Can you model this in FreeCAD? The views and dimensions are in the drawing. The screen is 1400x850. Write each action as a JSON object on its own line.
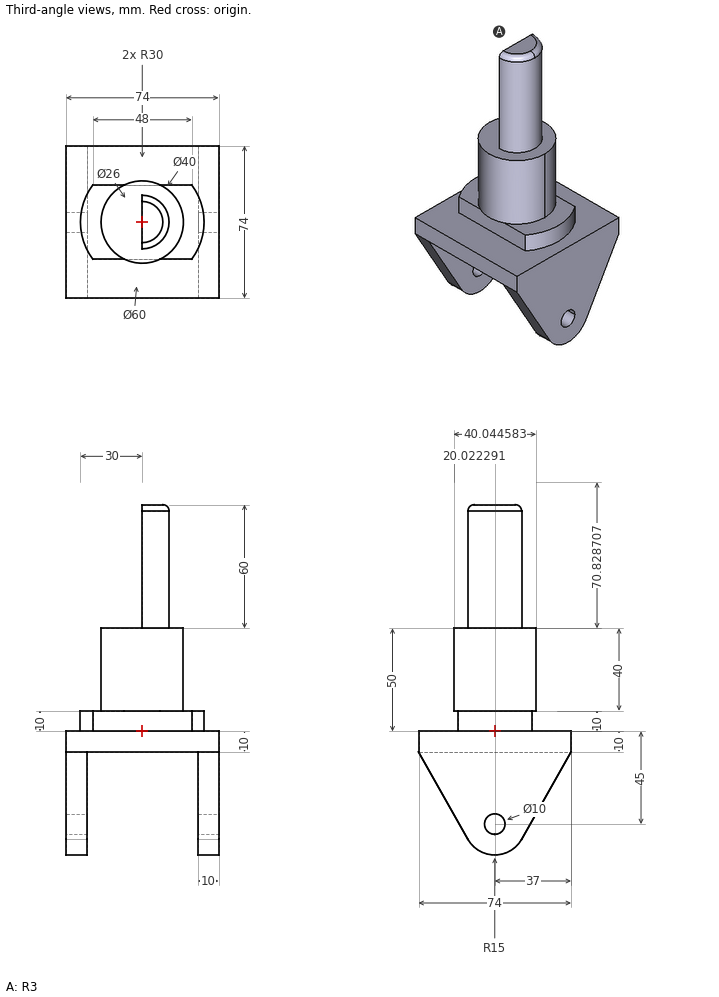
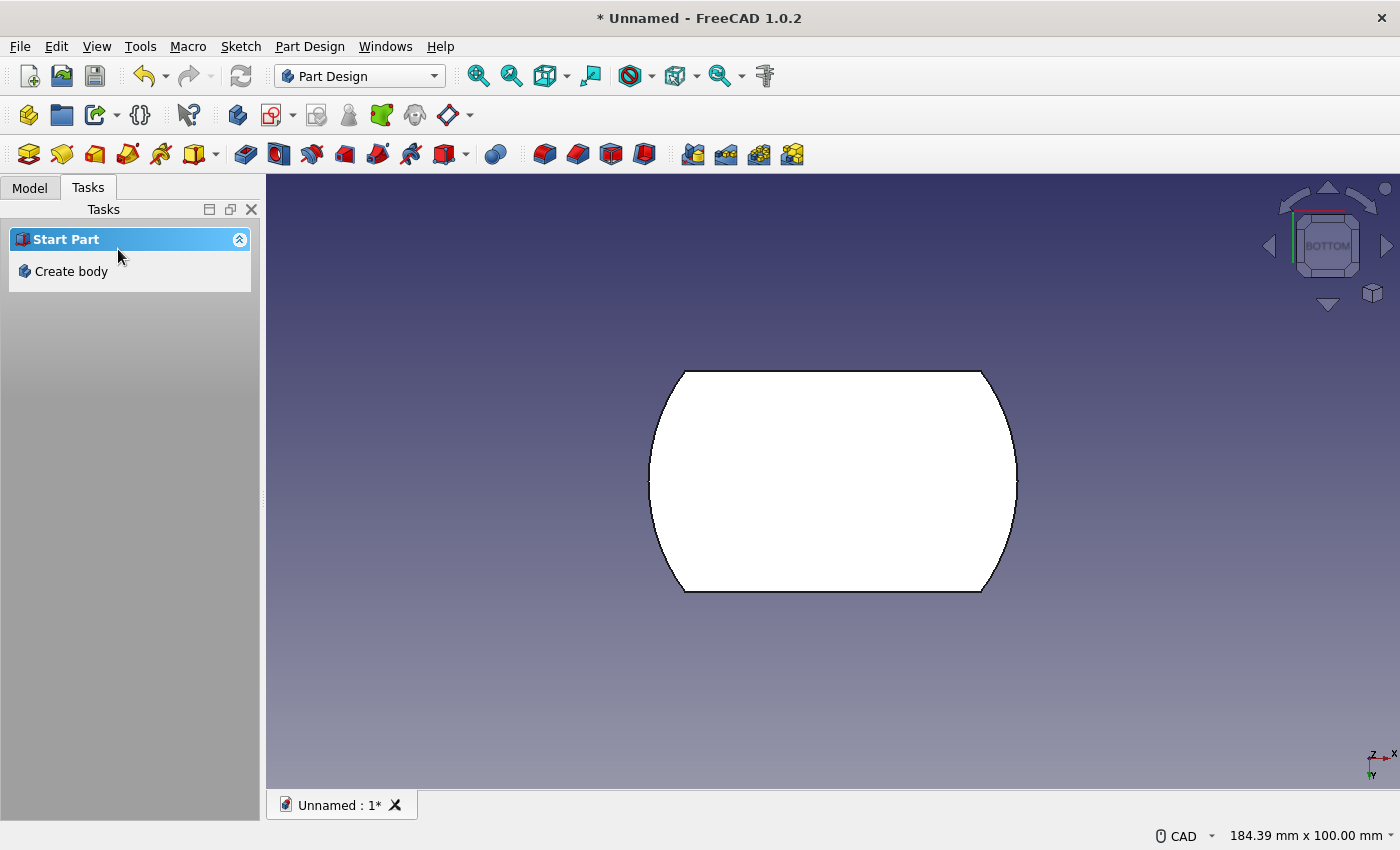
{"action": "key", "text": "v f"}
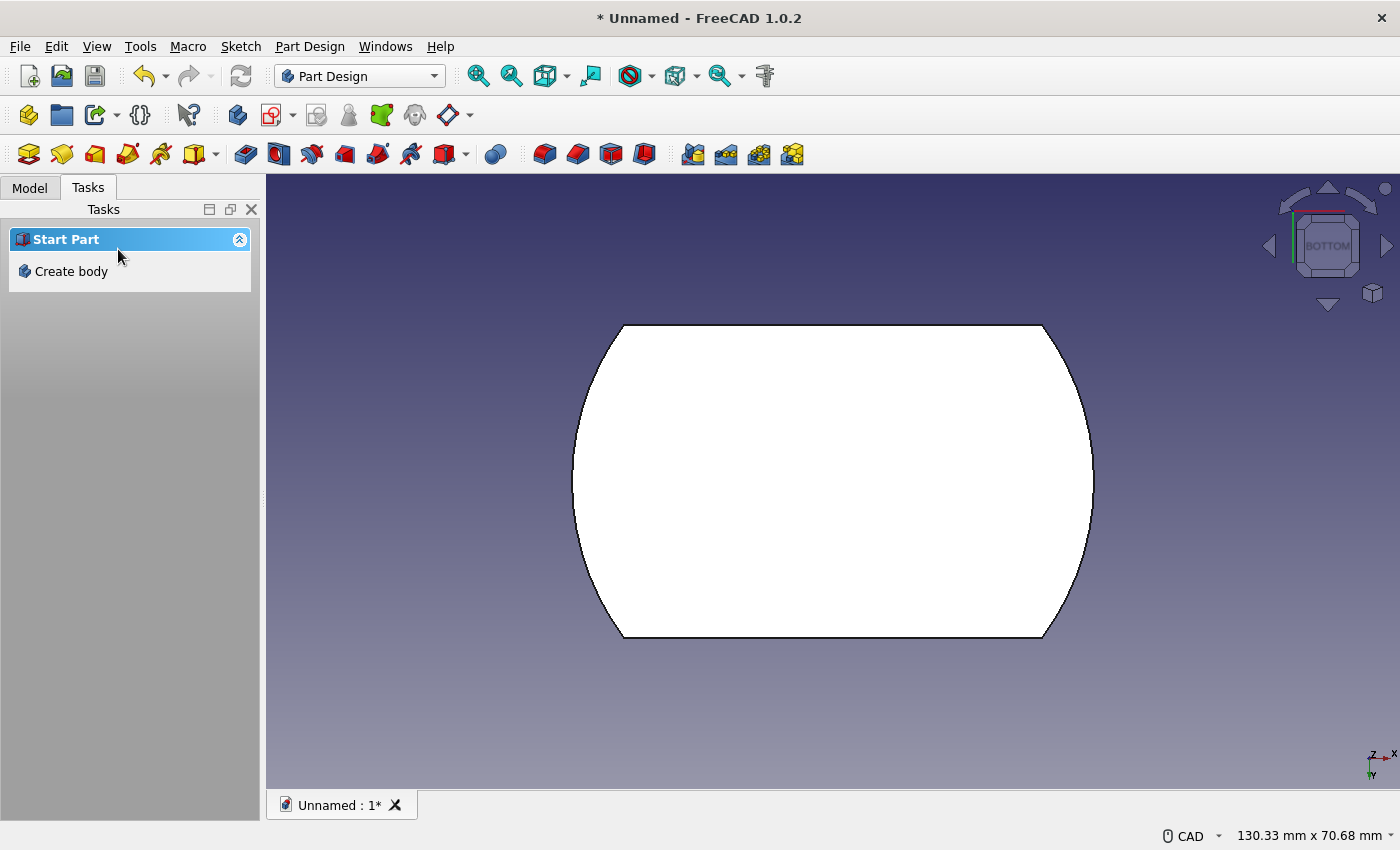
{"action": "key", "text": "0"}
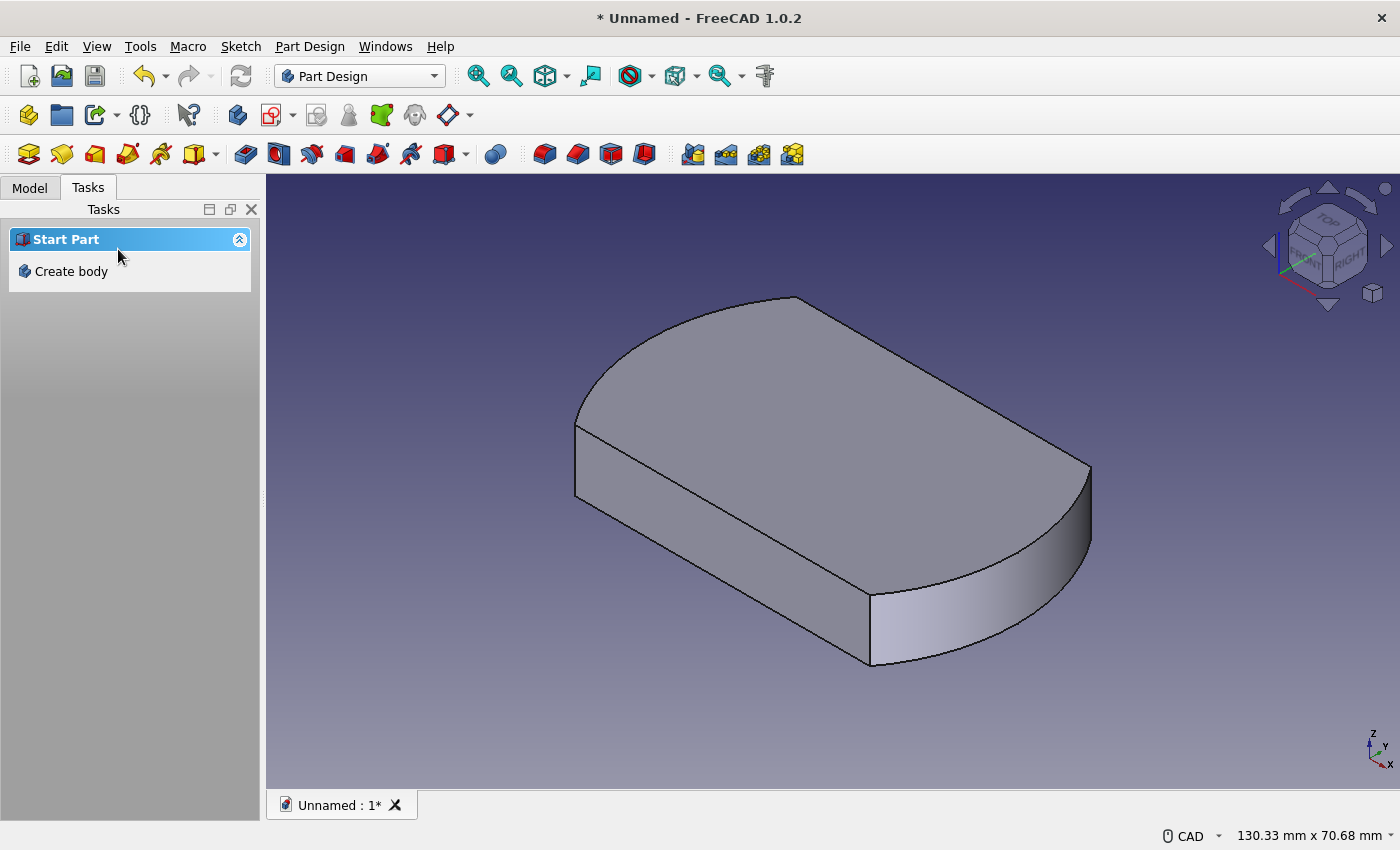
{"action": "left_click", "coordinate": [886, 475]}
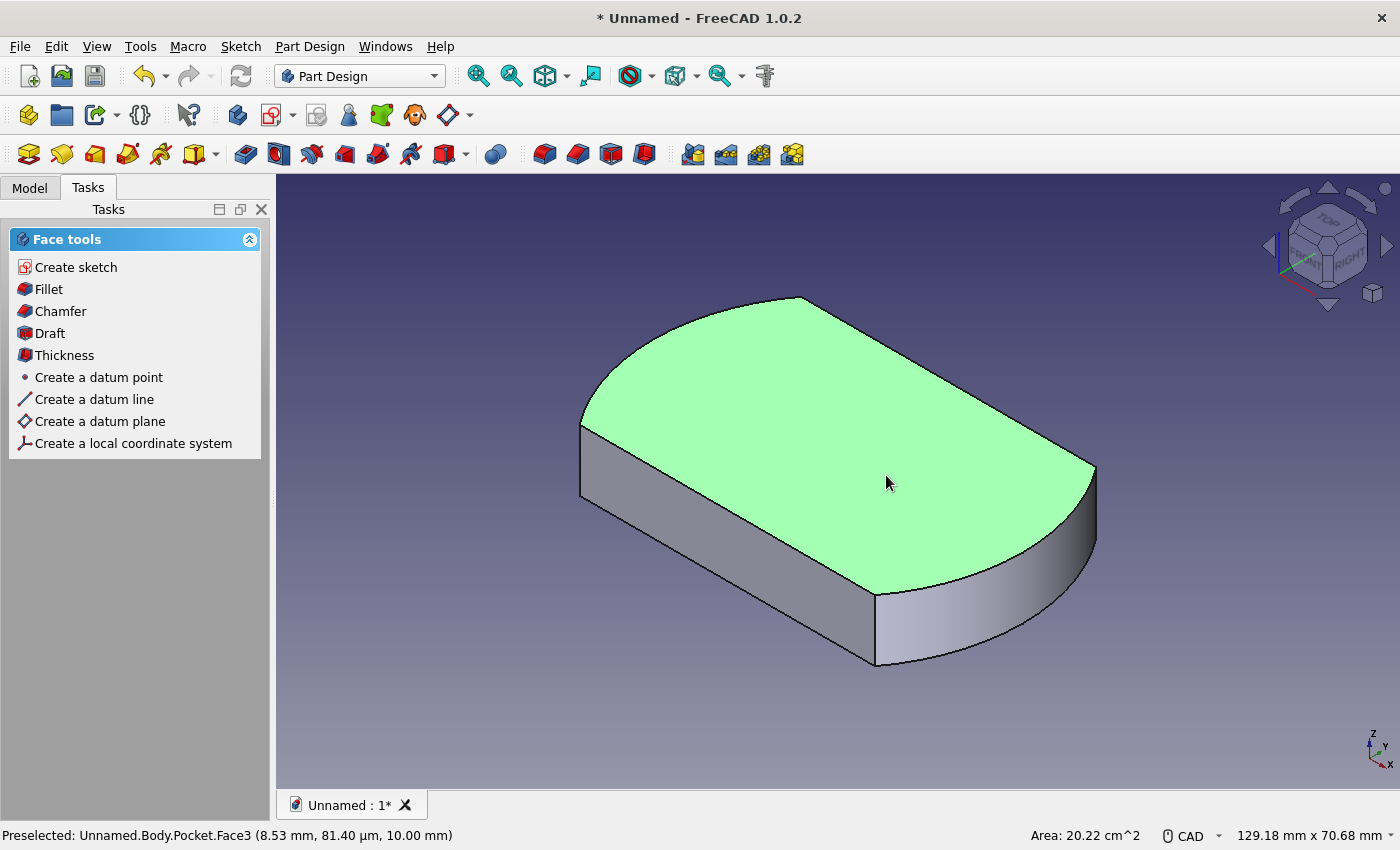
{"action": "left_click", "coordinate": [270, 116]}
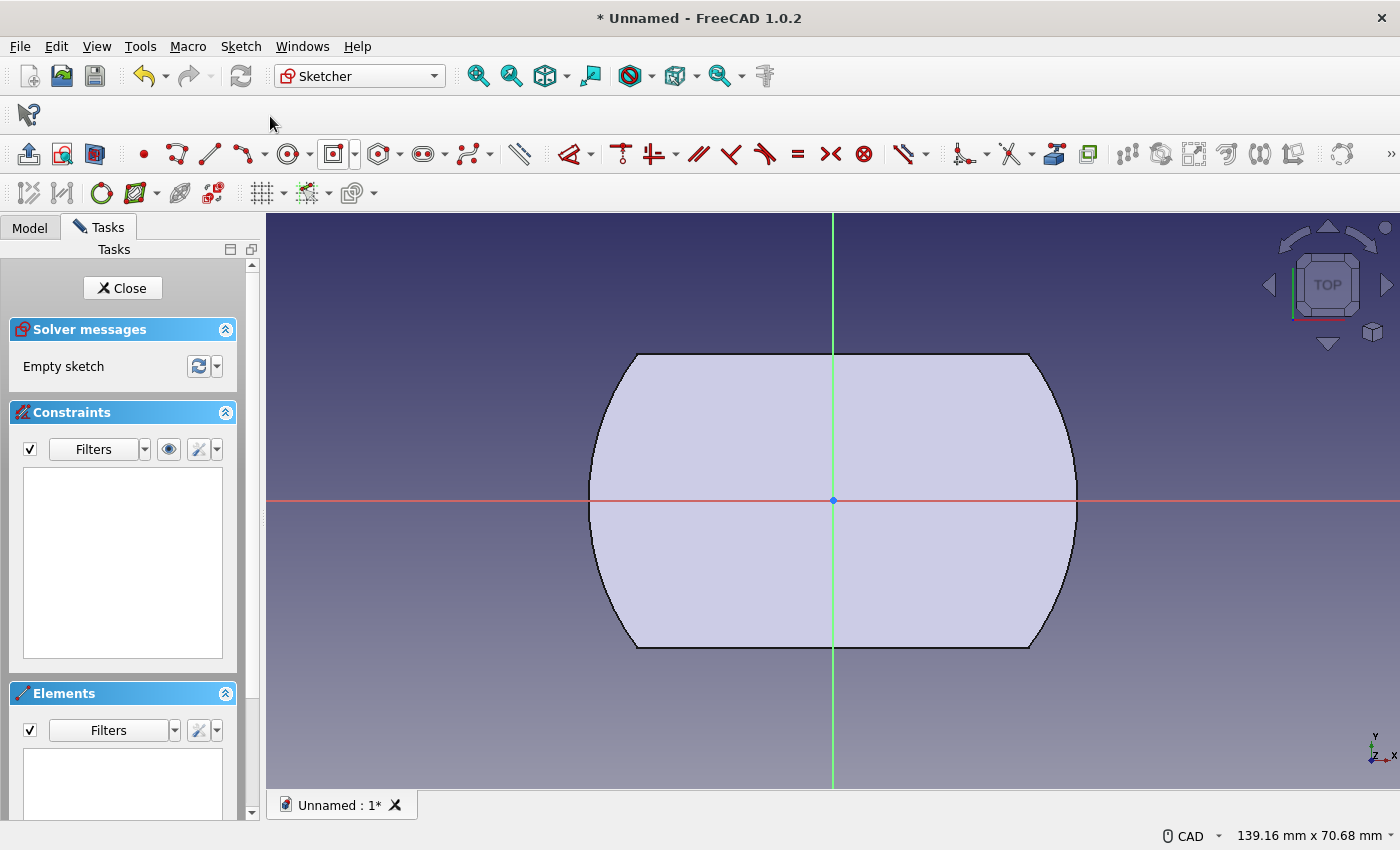
{"action": "left_click", "coordinate": [288, 154]}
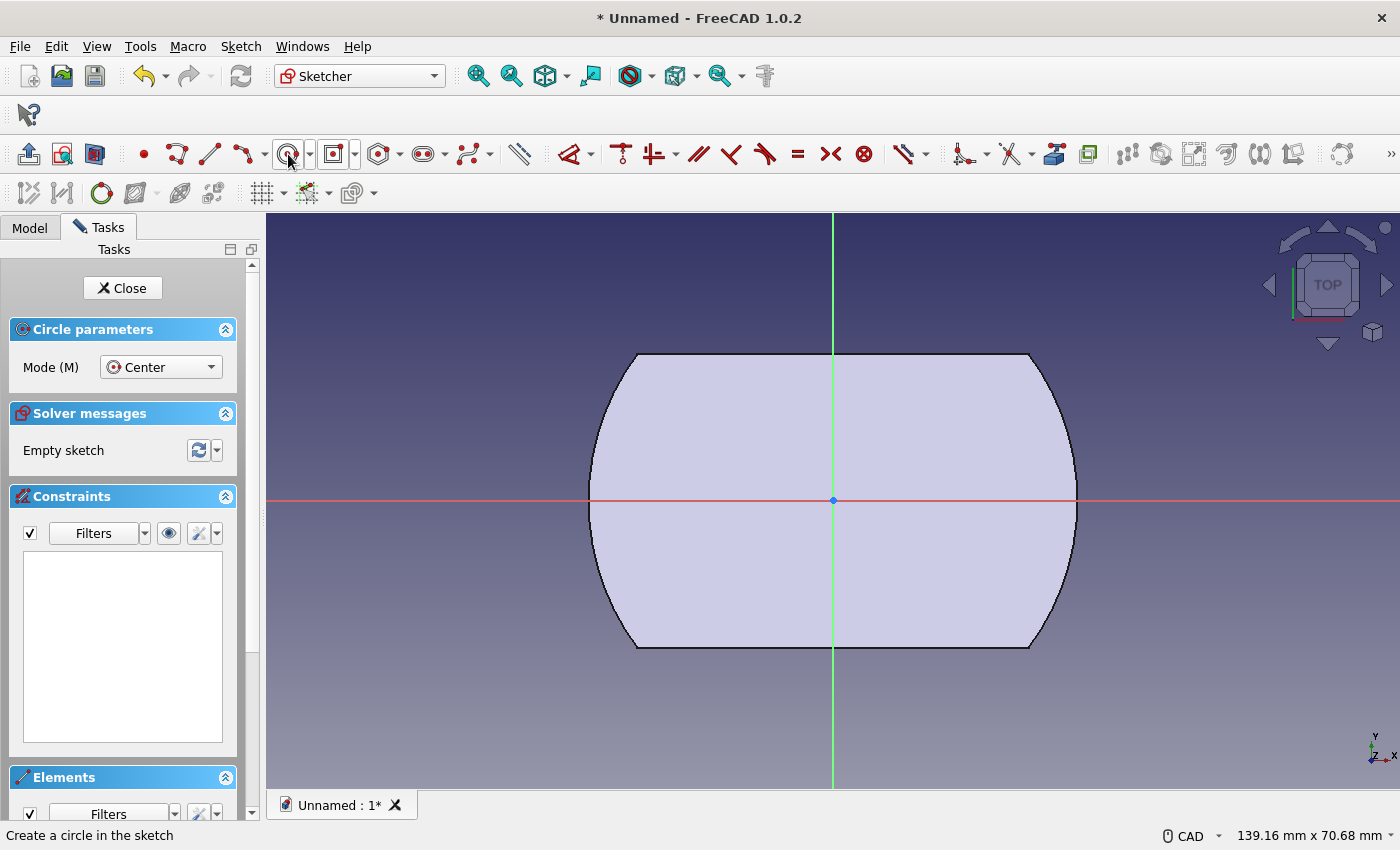
{"action": "left_click", "coordinate": [833, 501]}
{"action": "mouse_move", "coordinate": [948, 386]}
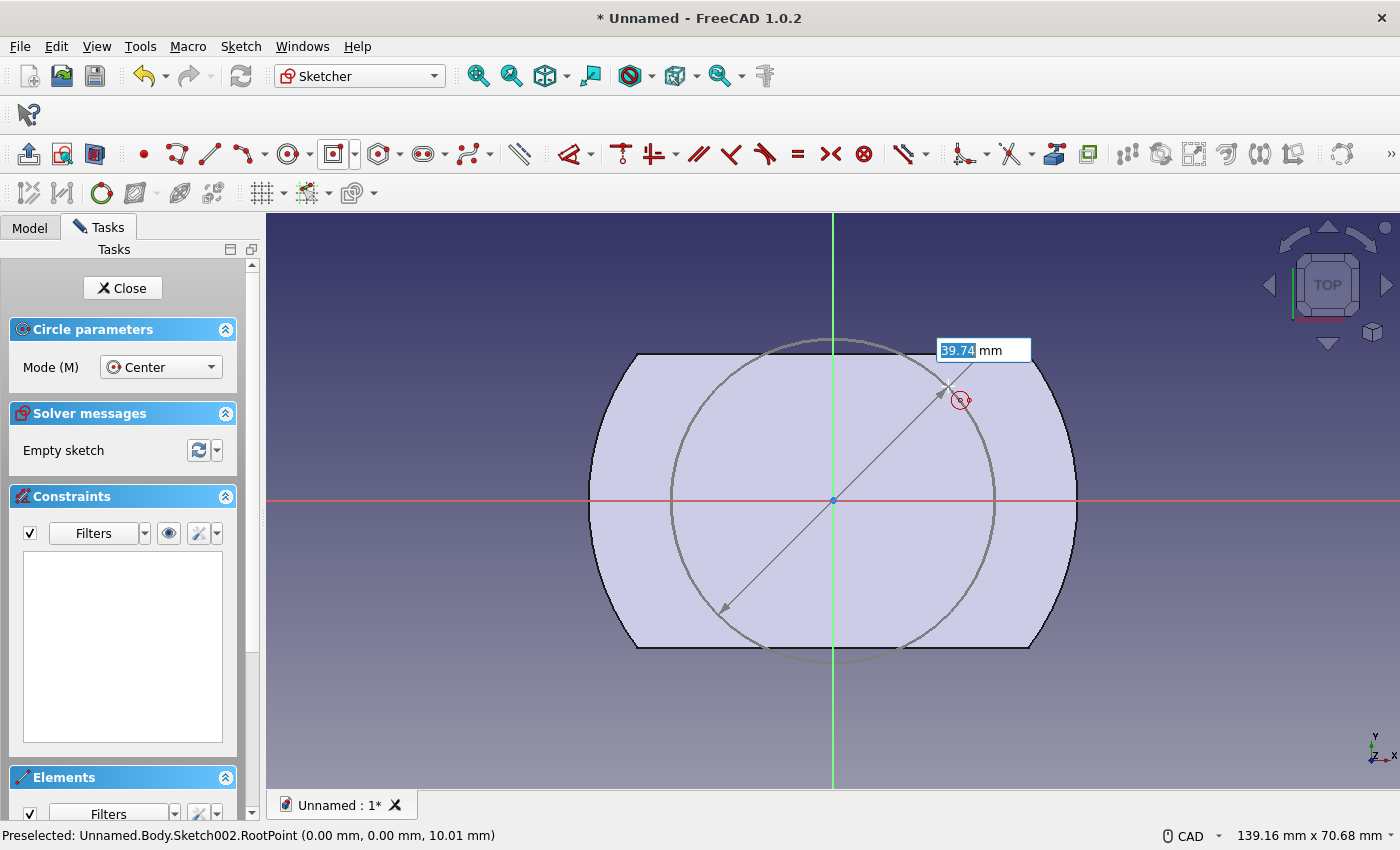
{"action": "type", "text": "40"}
{"action": "key", "text": "Return"}
{"action": "key", "text": "Escape"}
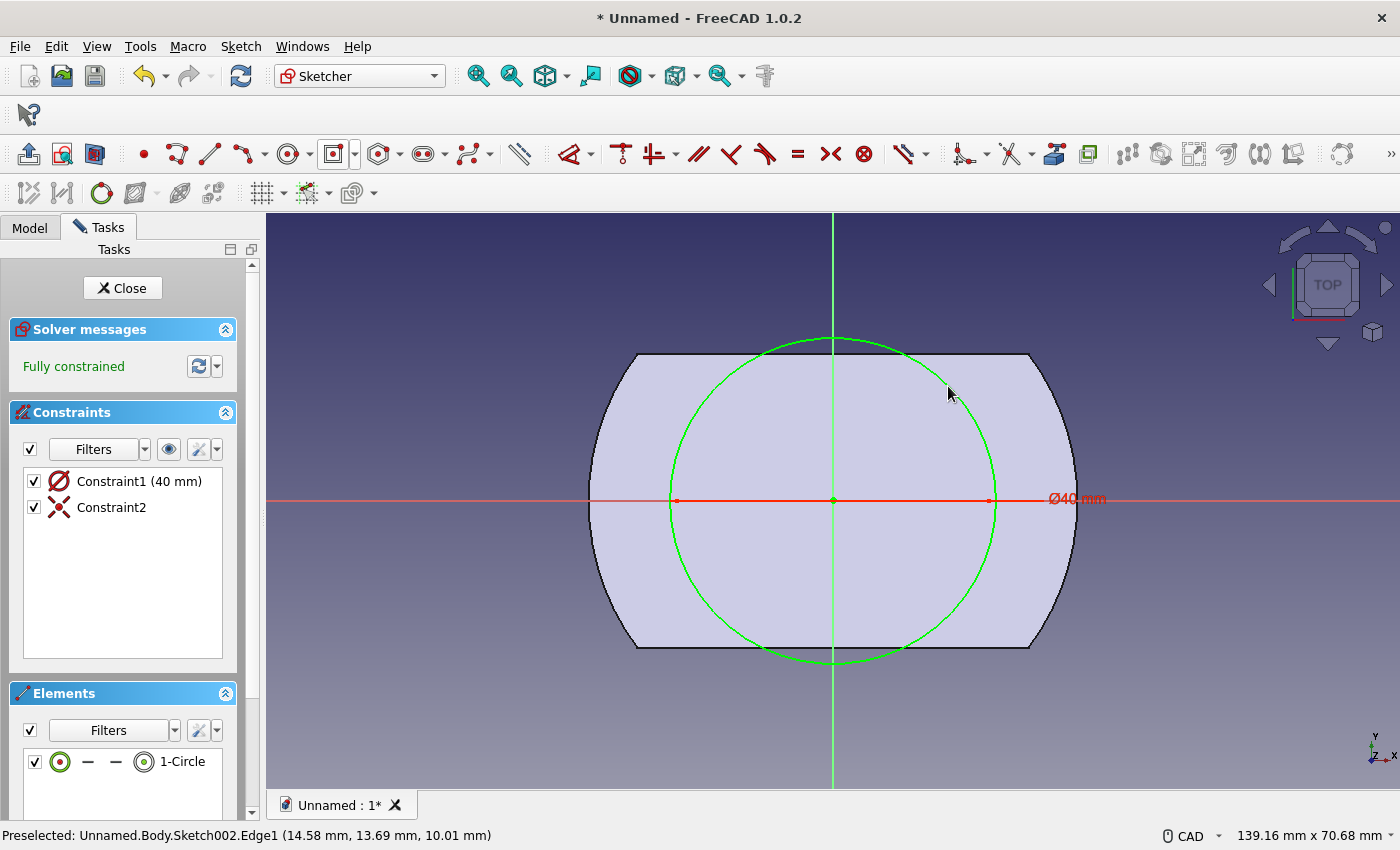
{"action": "left_click", "coordinate": [123, 288]}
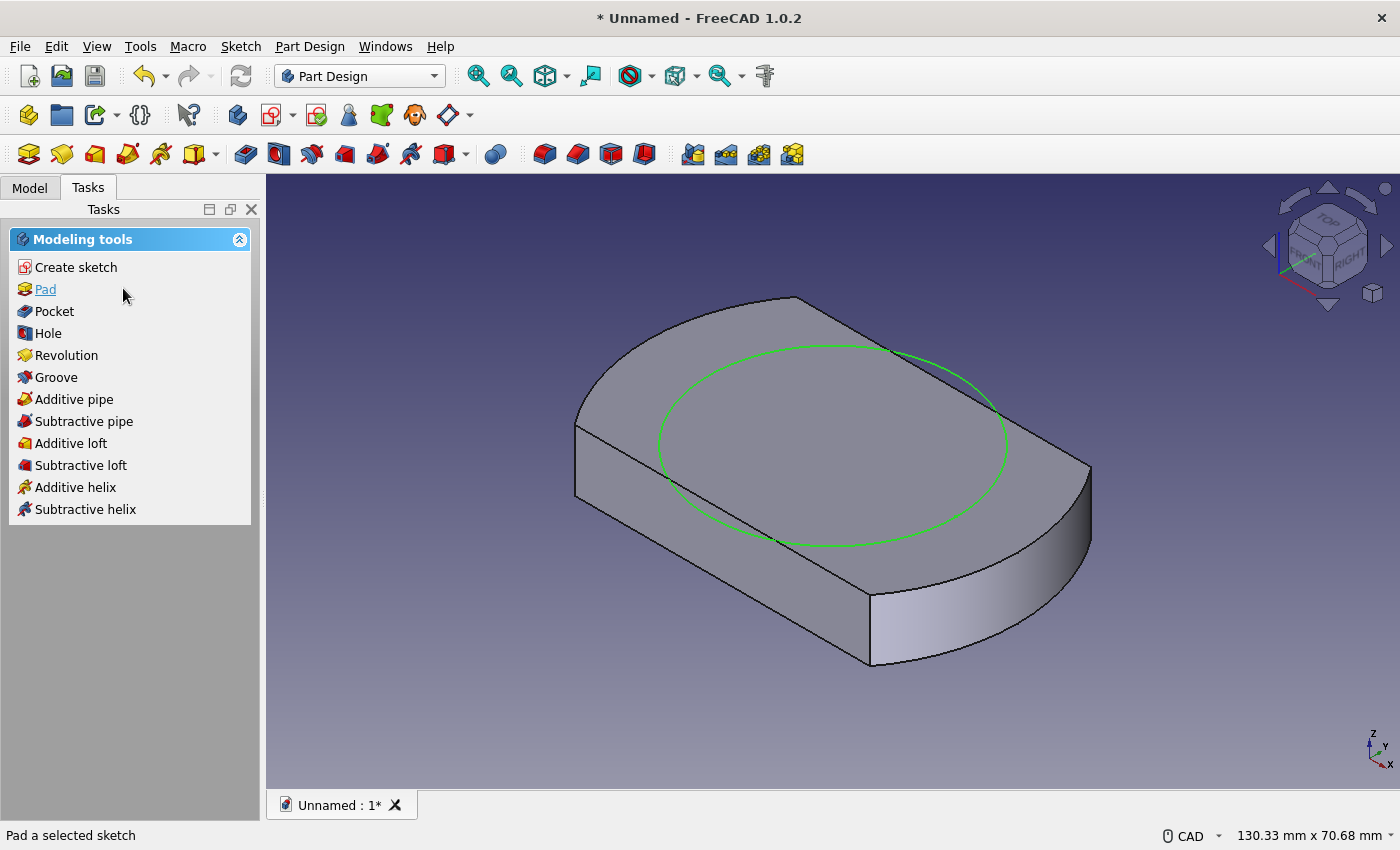
{"action": "left_click", "coordinate": [29, 154]}